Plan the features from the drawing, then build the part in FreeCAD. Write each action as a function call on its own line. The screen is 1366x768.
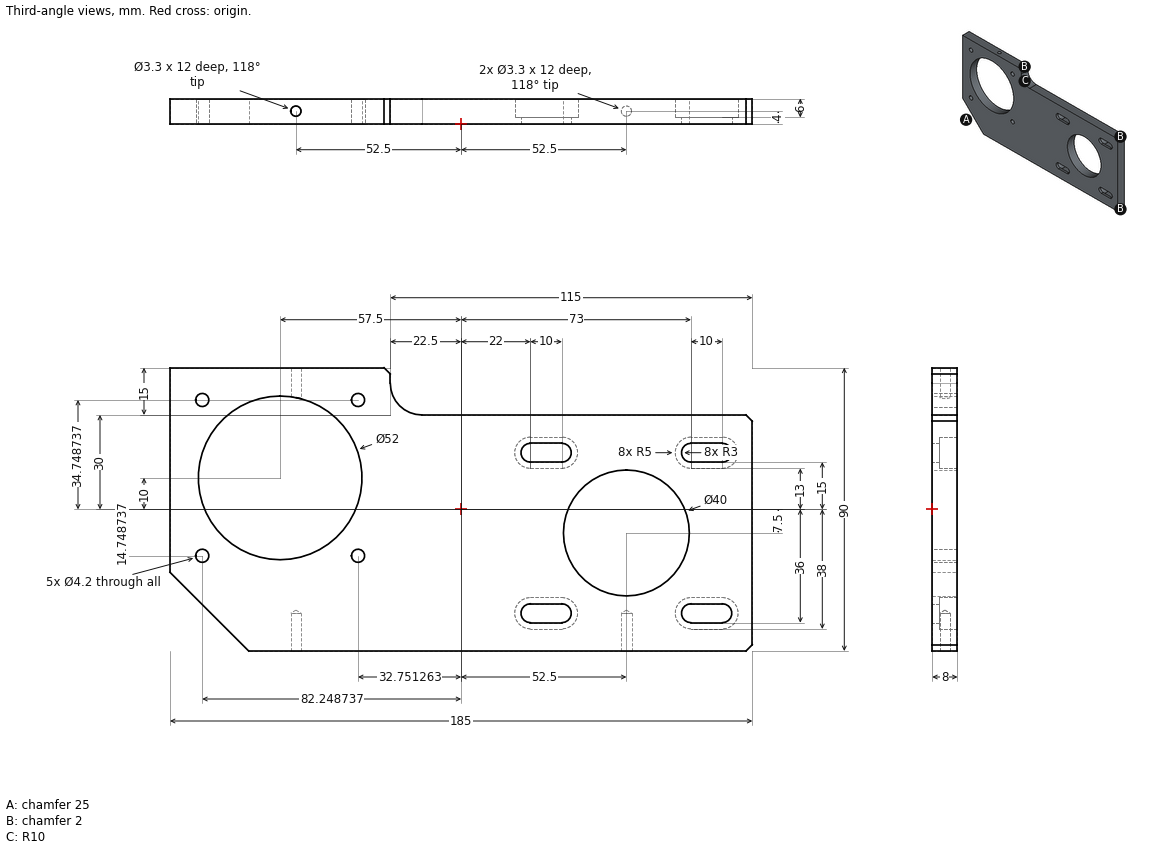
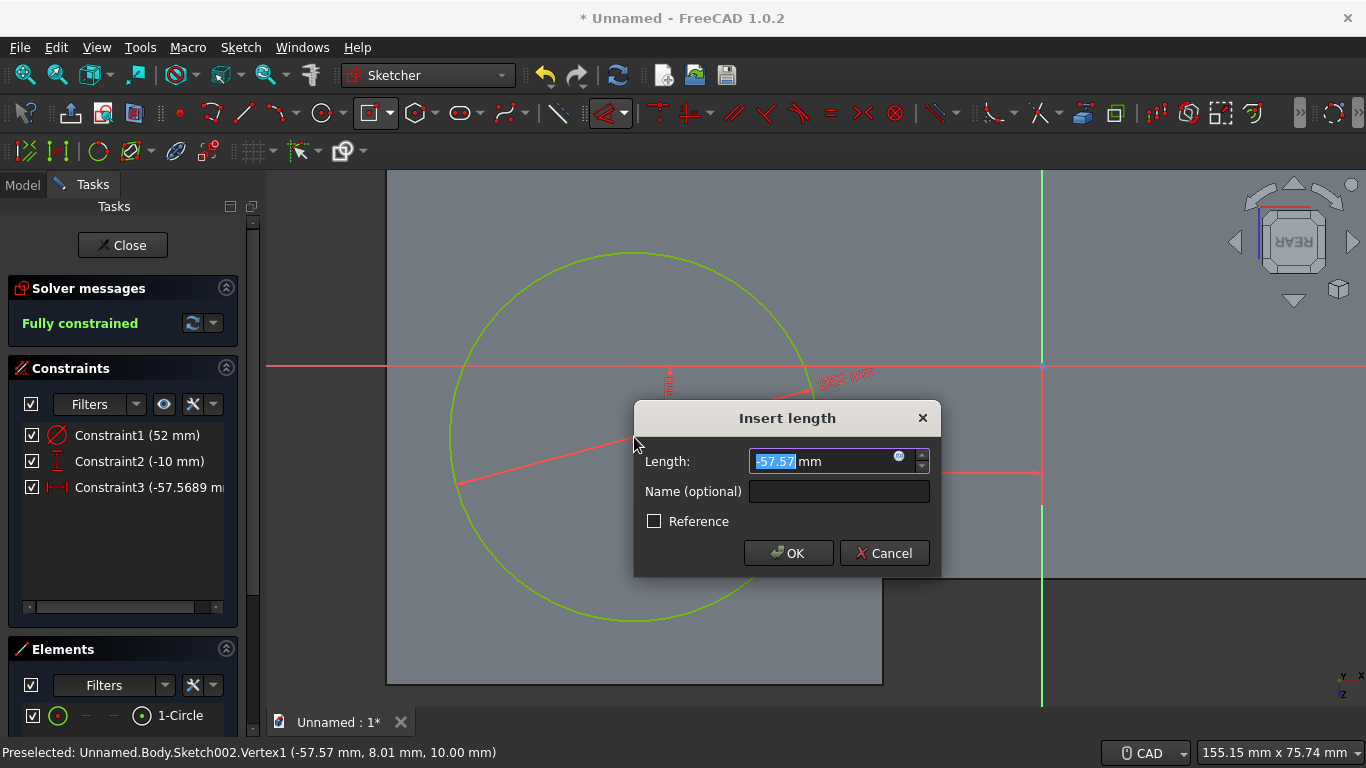
text(-57.5)
key(Return)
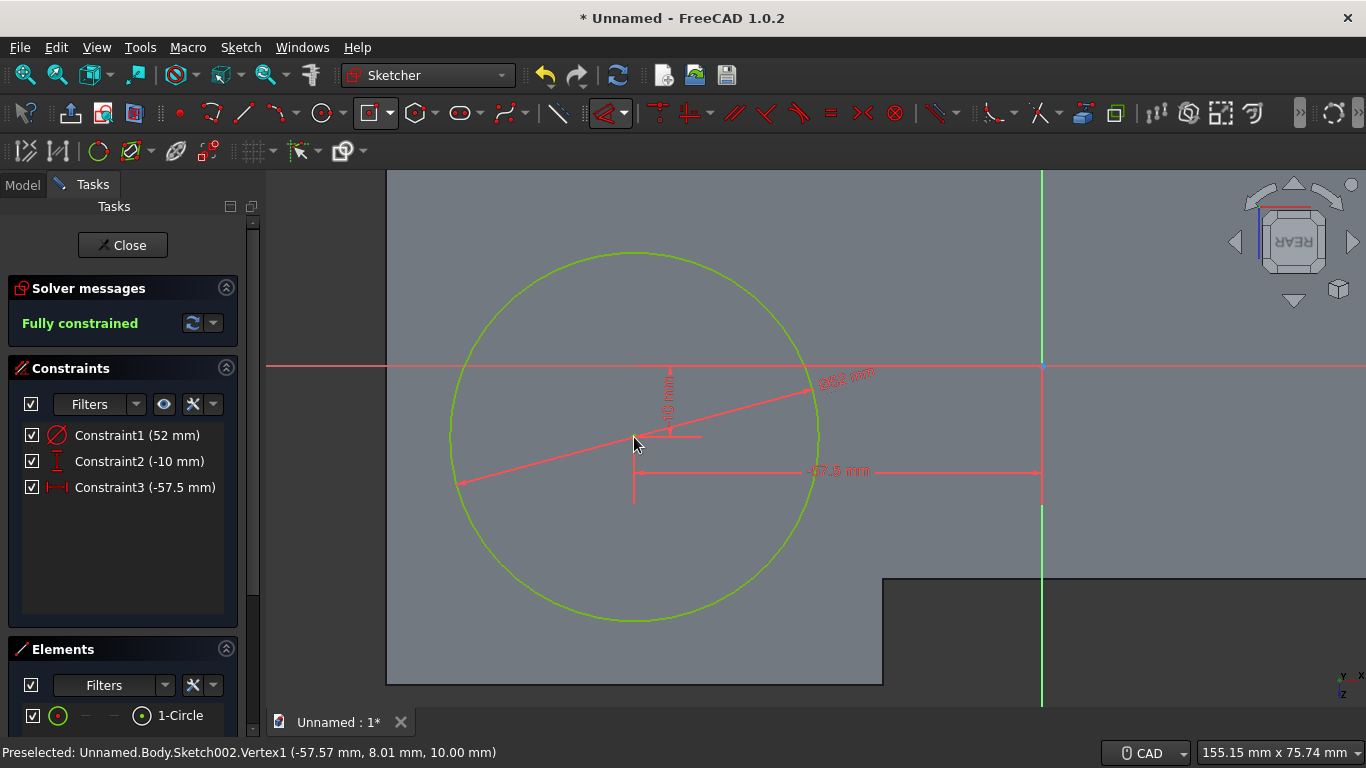
click(123, 245)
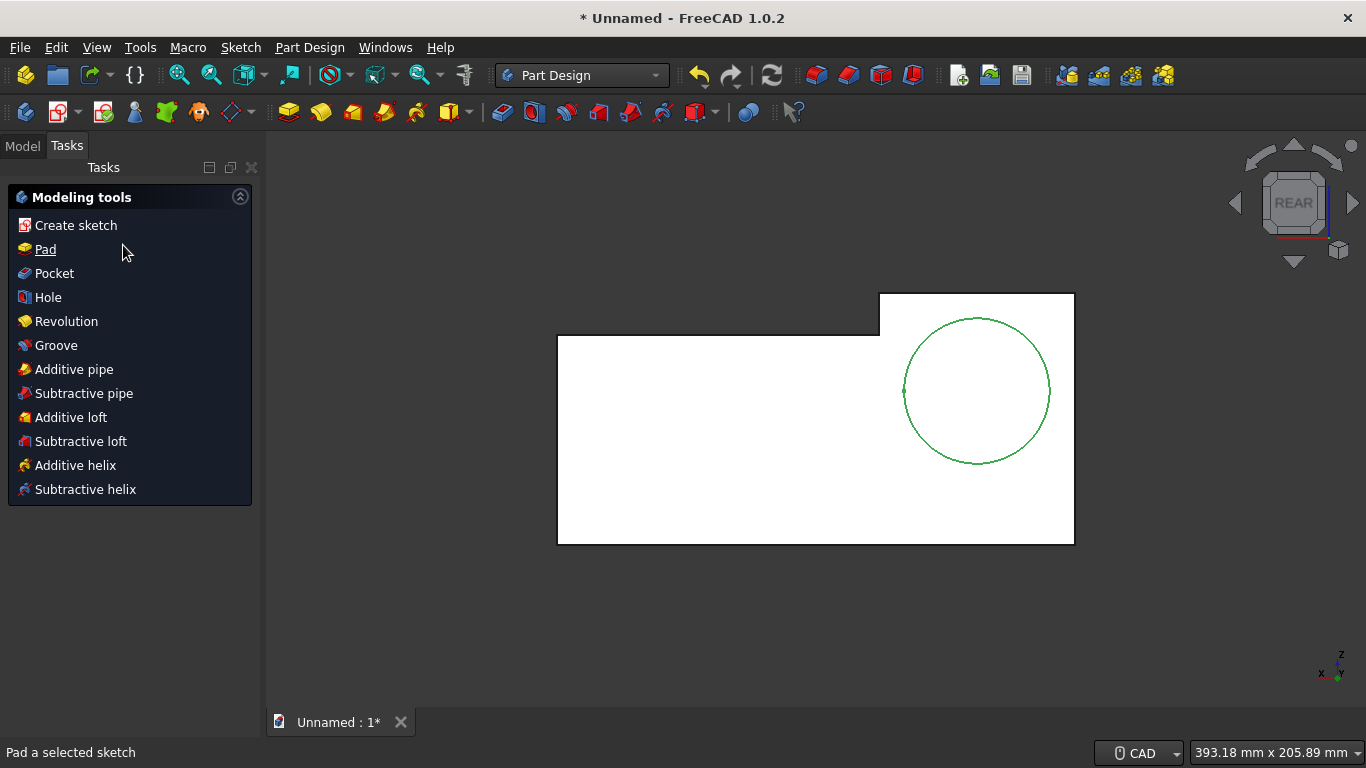
click(504, 112)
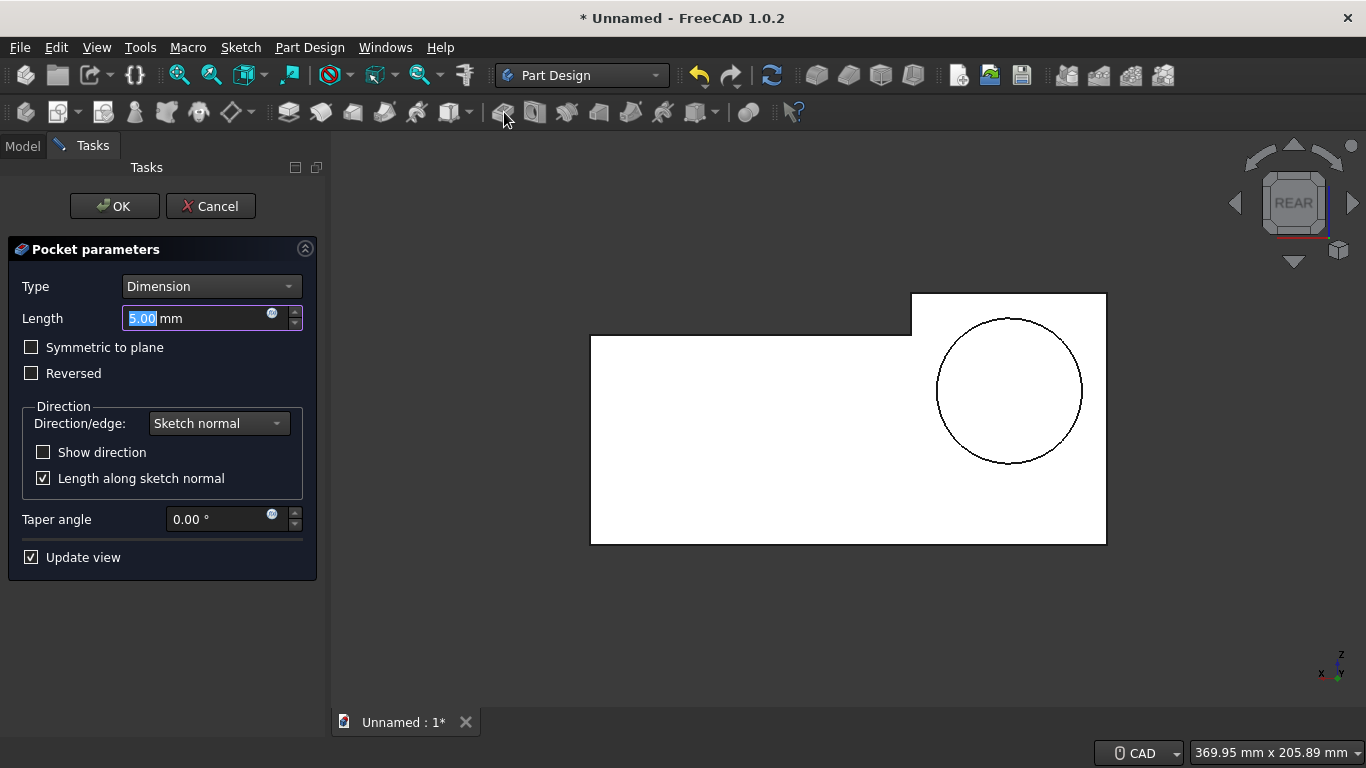
click(212, 286)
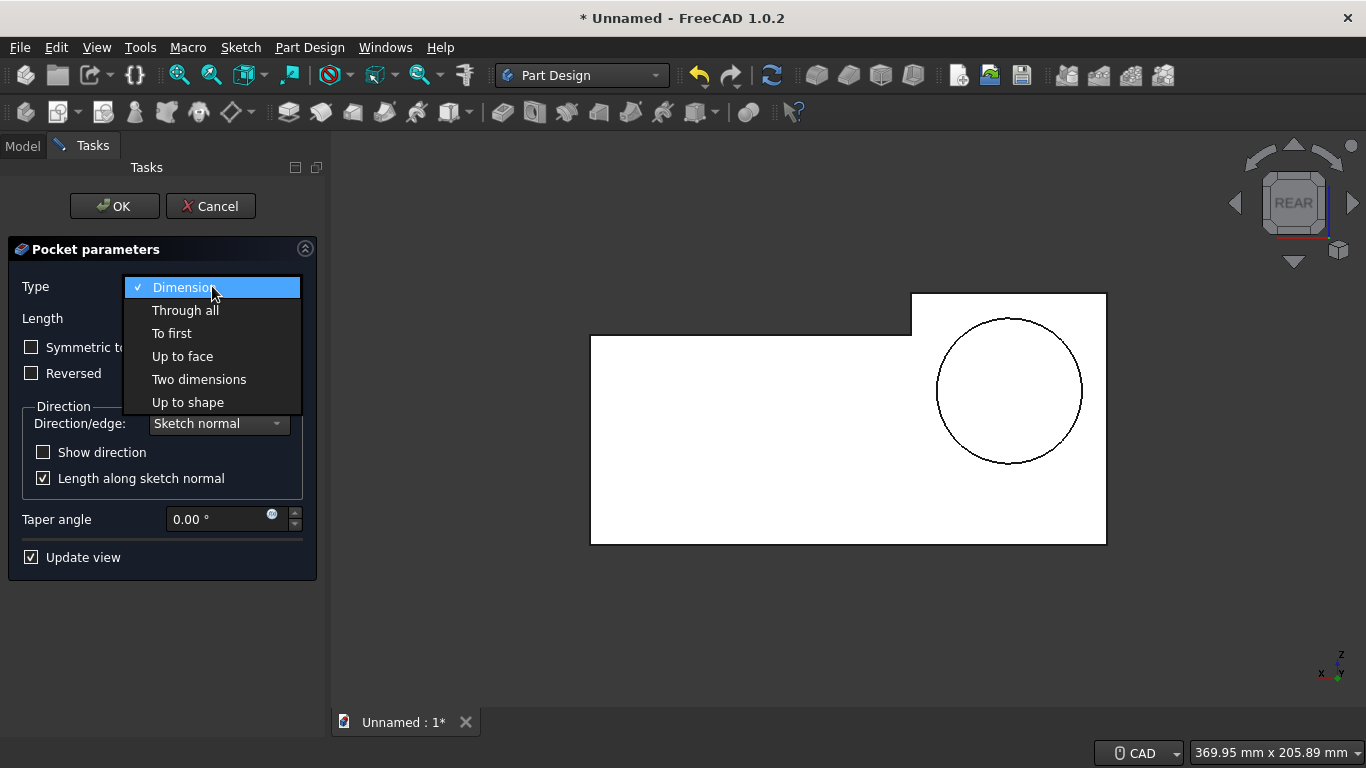
click(212, 310)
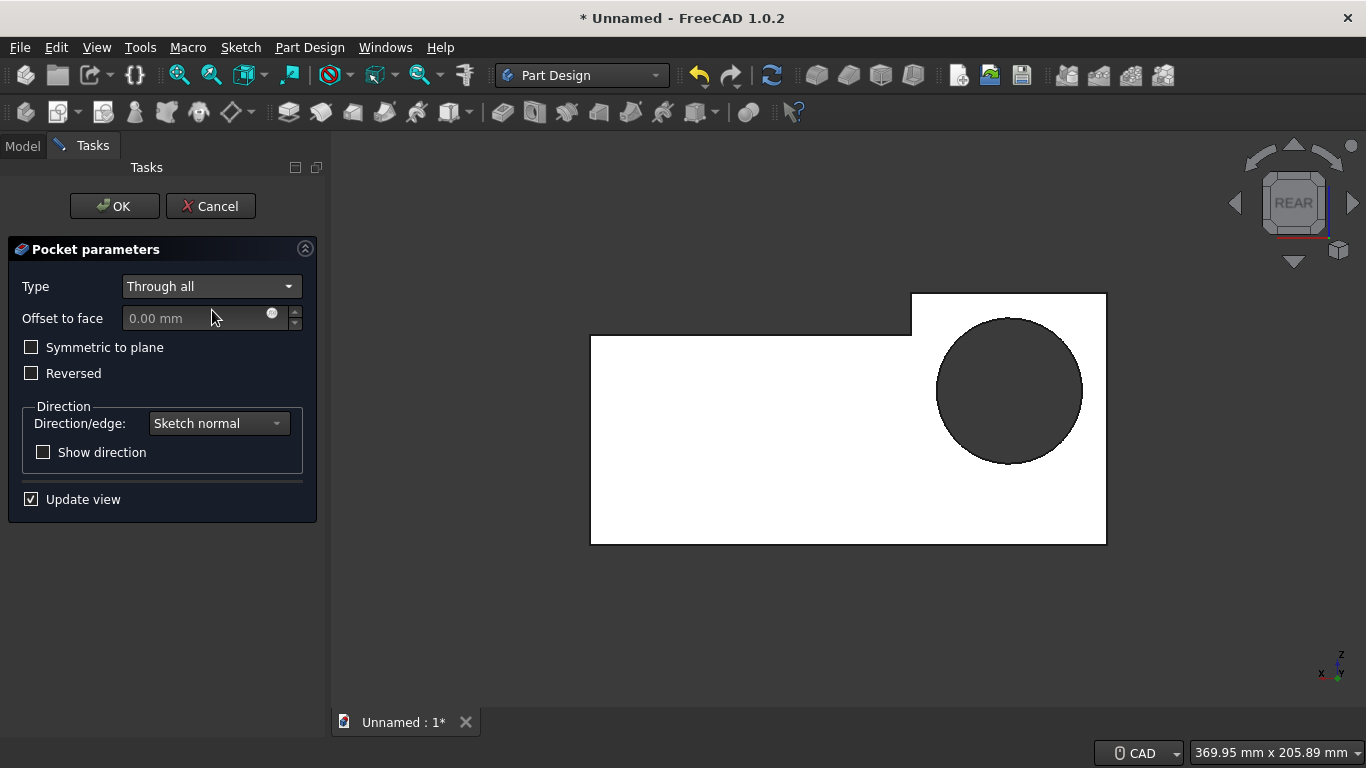
click(115, 206)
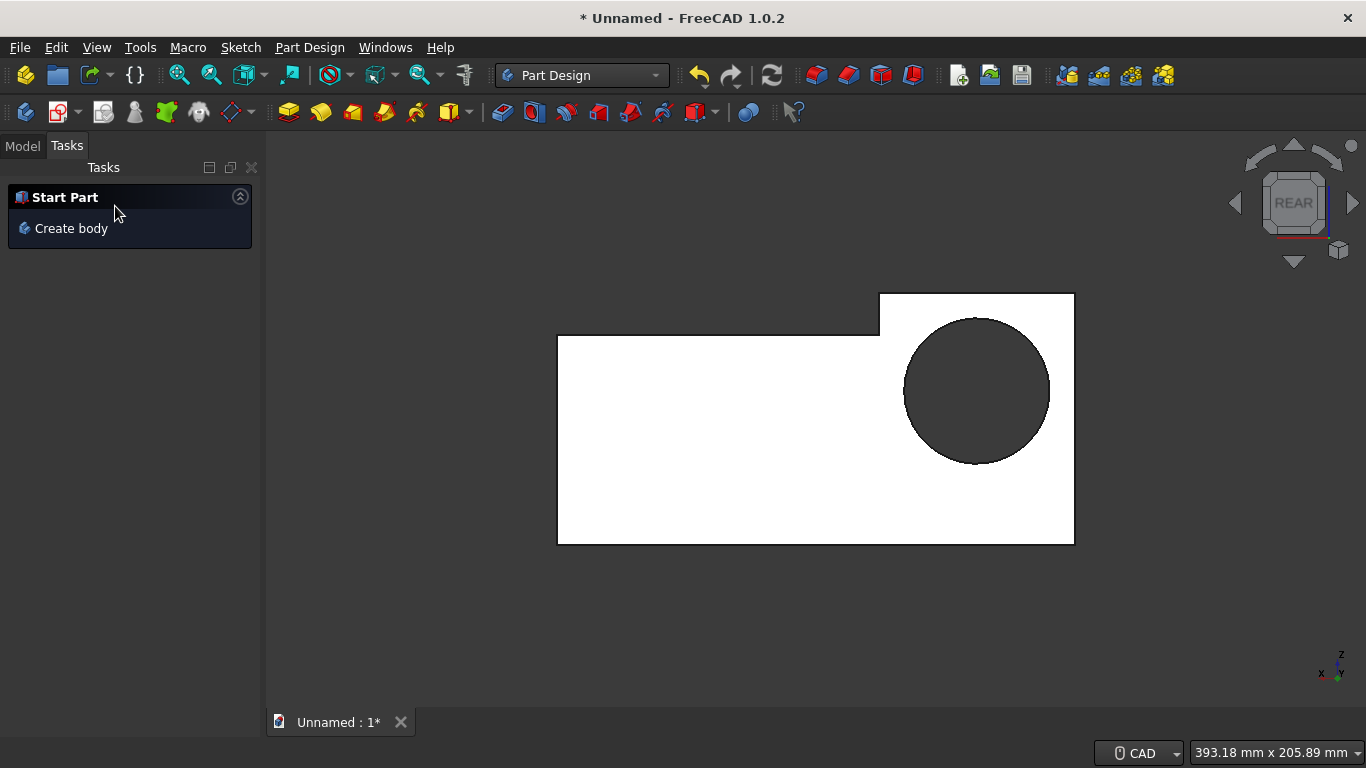
click(668, 454)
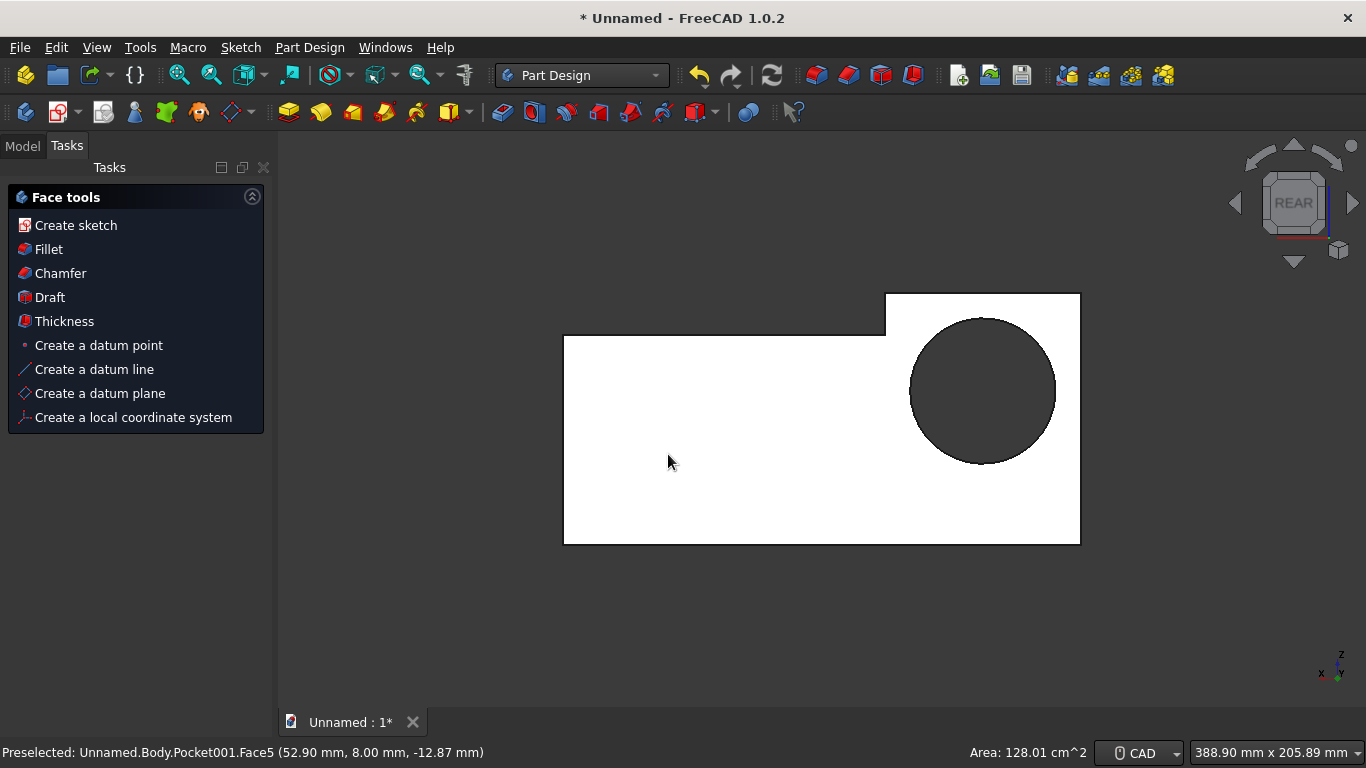
click(58, 112)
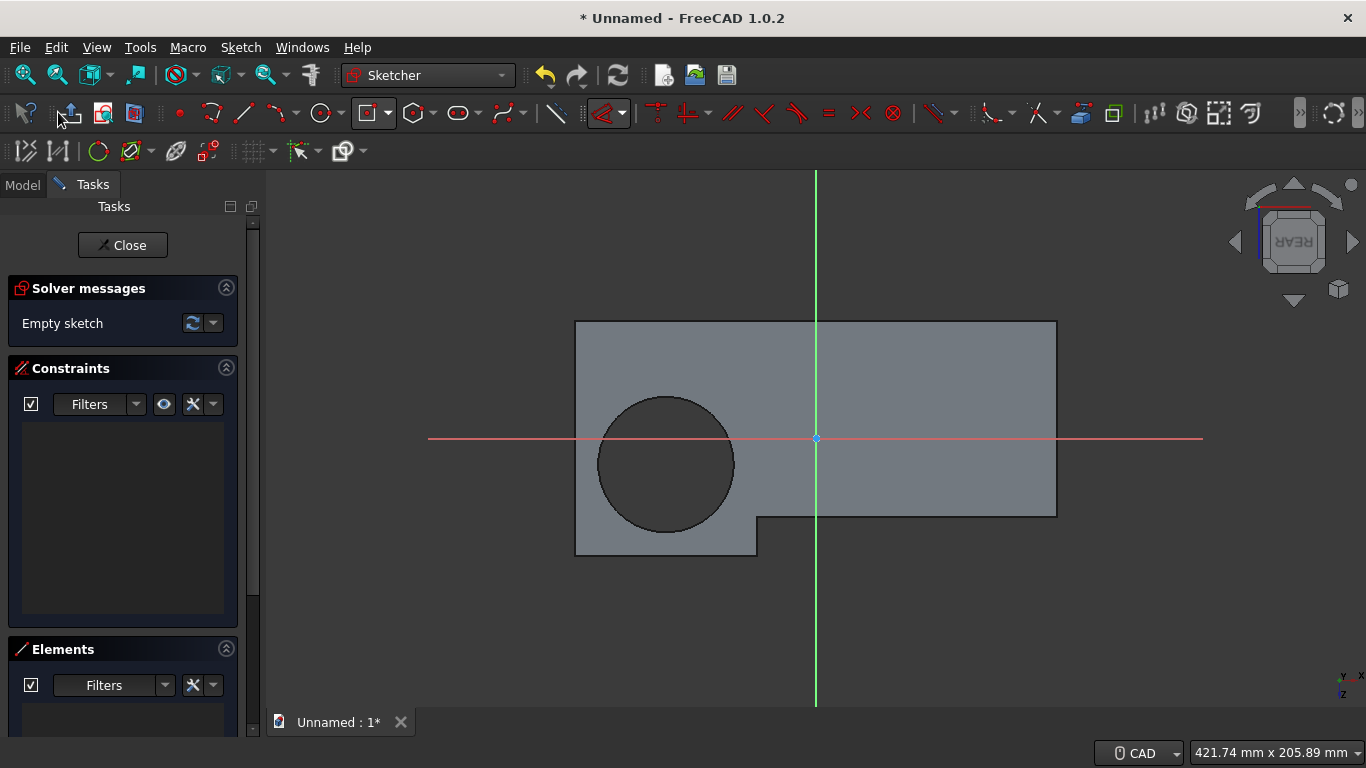
scroll(672, 486, up, 4)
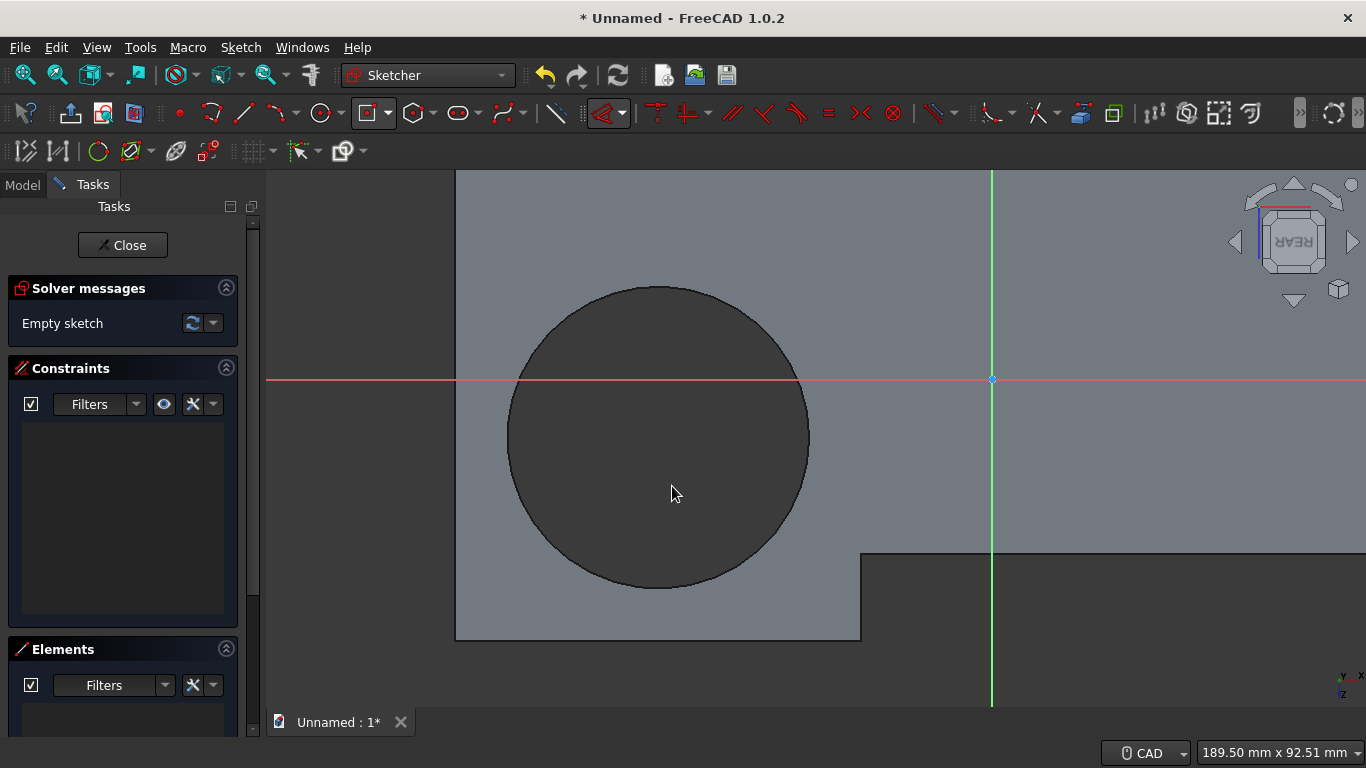
key(g)
key(c)